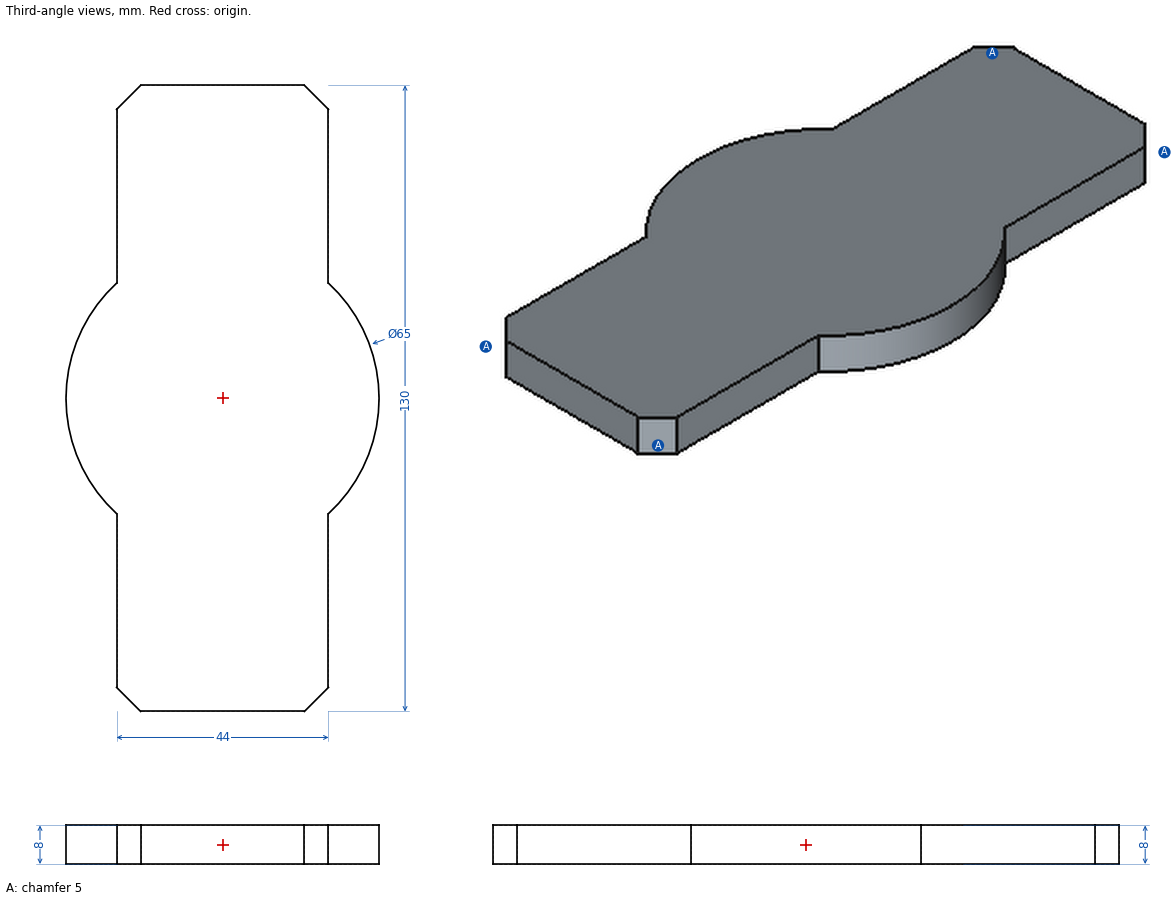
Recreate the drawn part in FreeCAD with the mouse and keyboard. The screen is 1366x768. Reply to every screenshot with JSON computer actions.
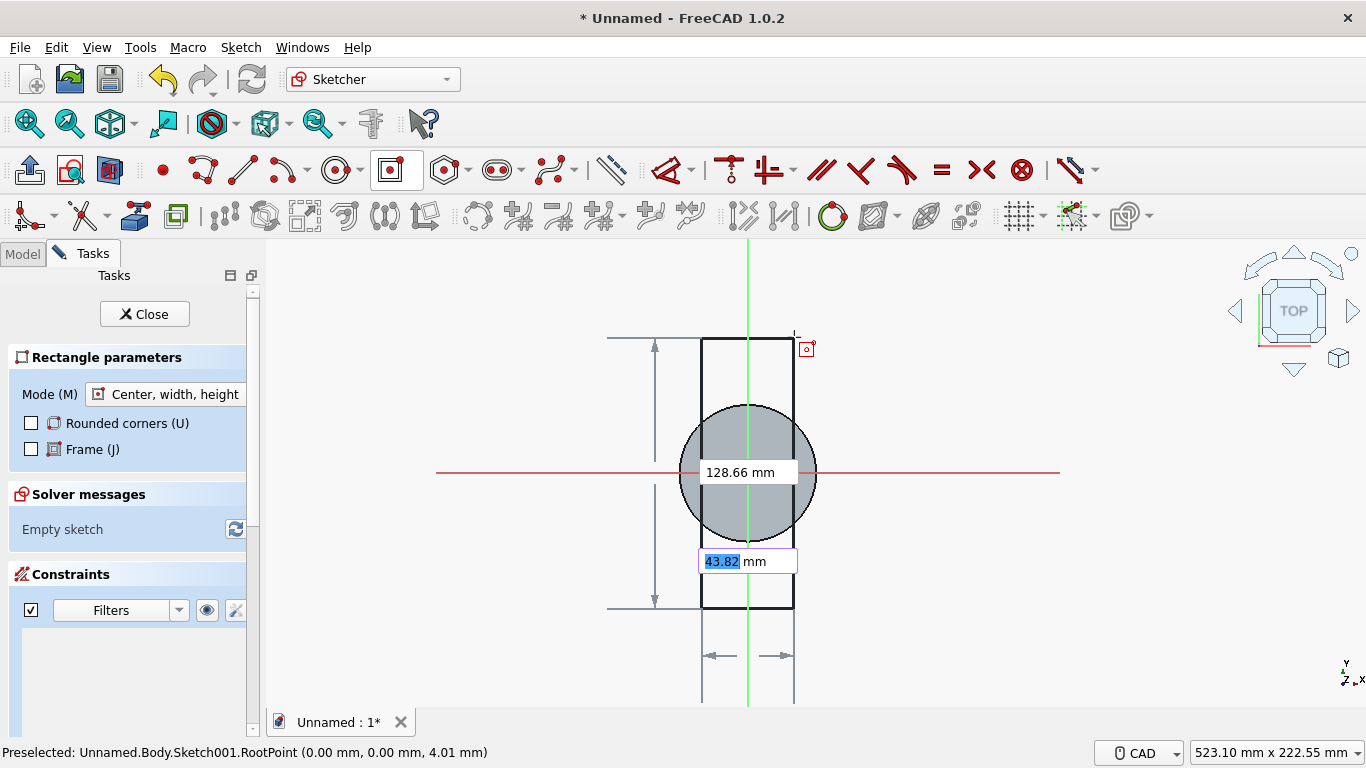
{"action": "type", "text": "44"}
{"action": "key", "text": "Tab"}
{"action": "type", "text": "130"}
{"action": "key", "text": "Return"}
{"action": "key", "text": "Escape"}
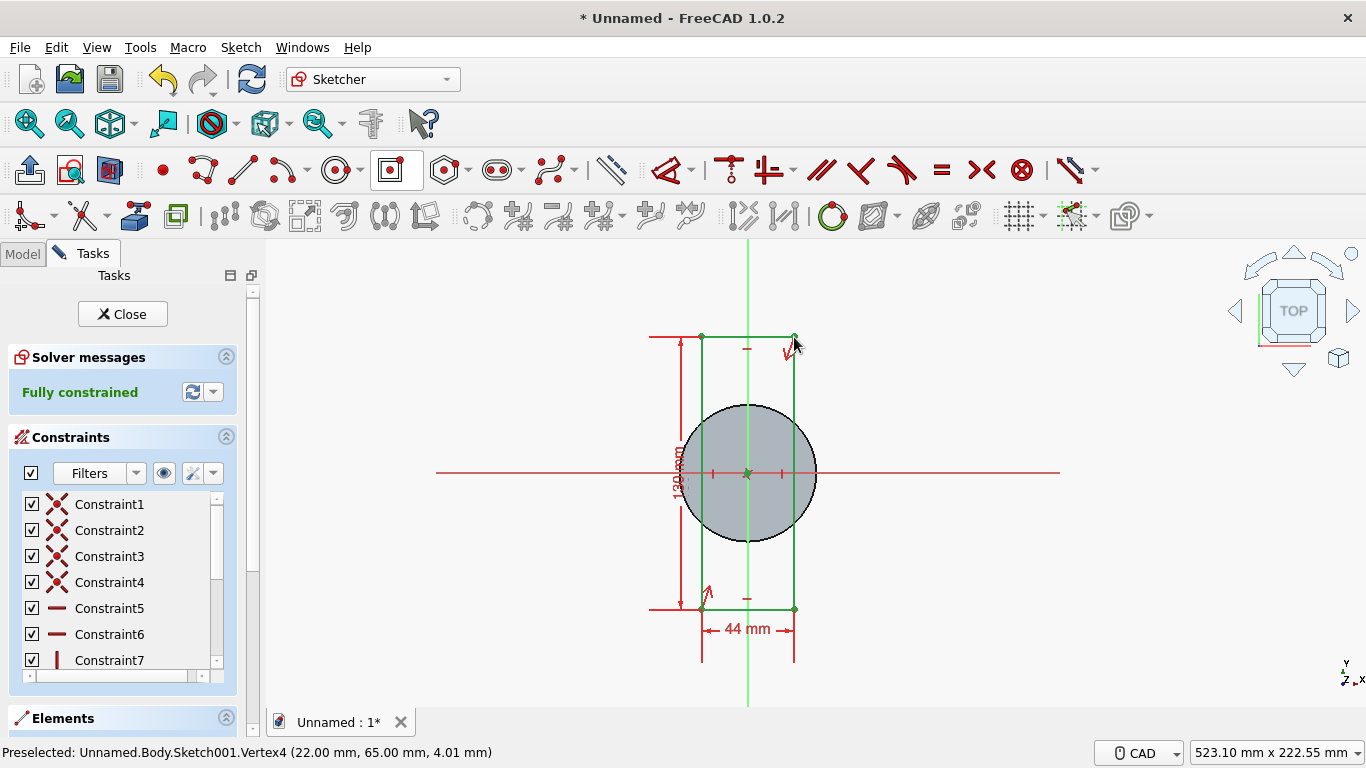
{"action": "left_click", "coordinate": [123, 314]}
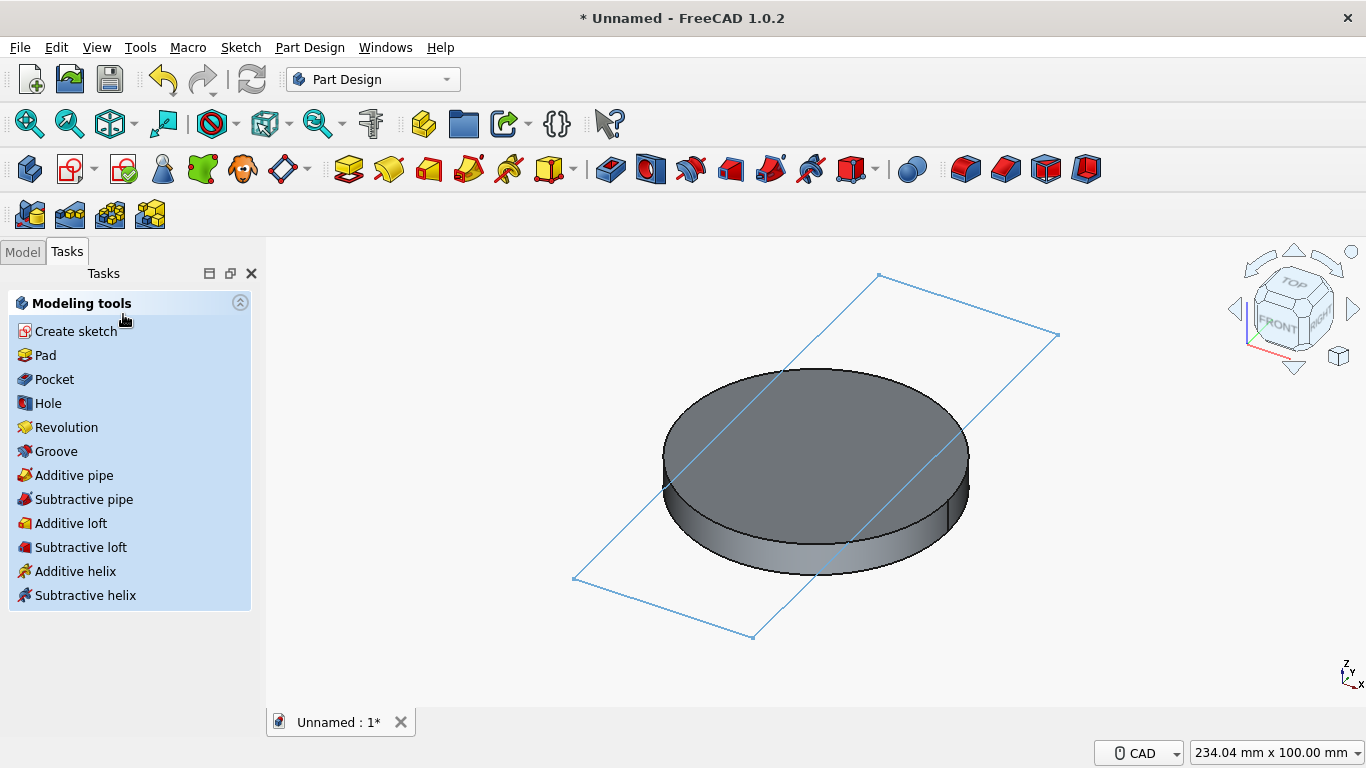
{"action": "left_click", "coordinate": [350, 170]}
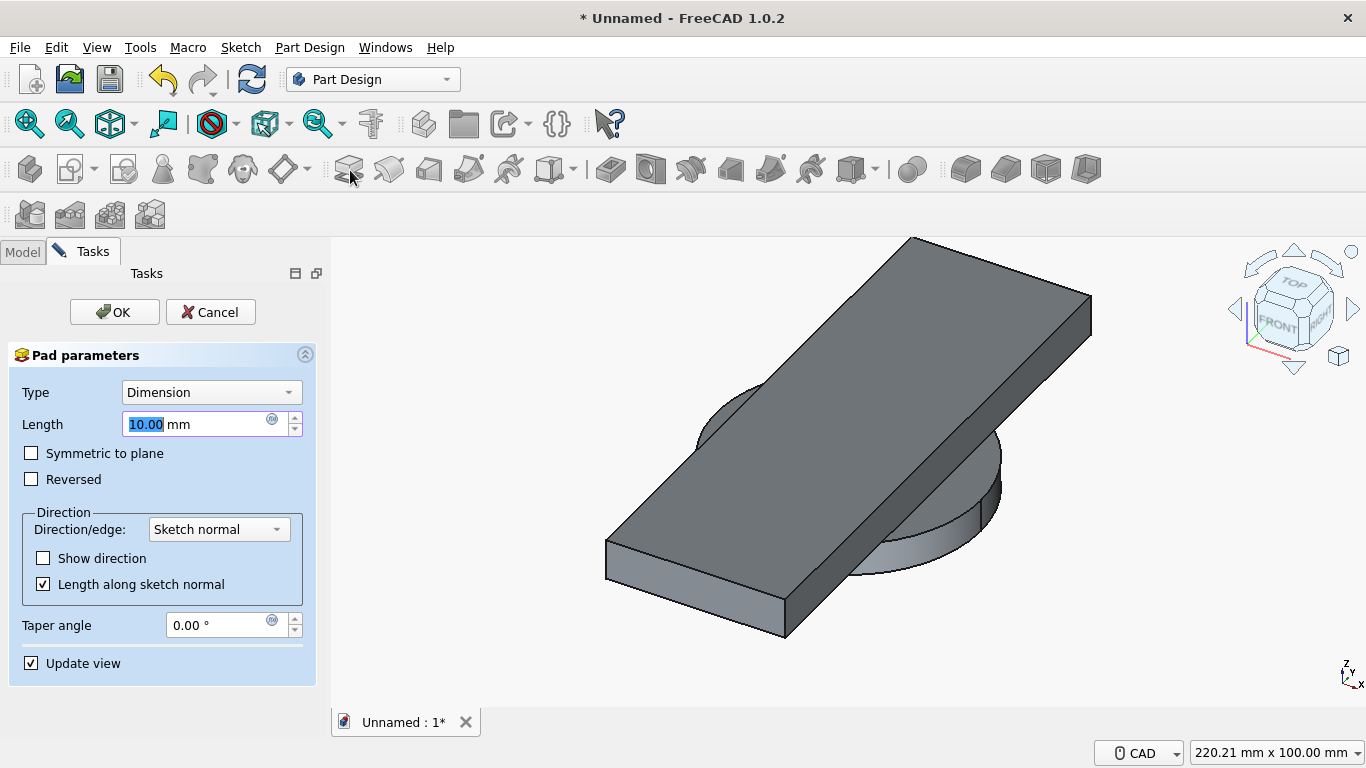
{"action": "type", "text": "8"}
{"action": "key", "text": "Tab"}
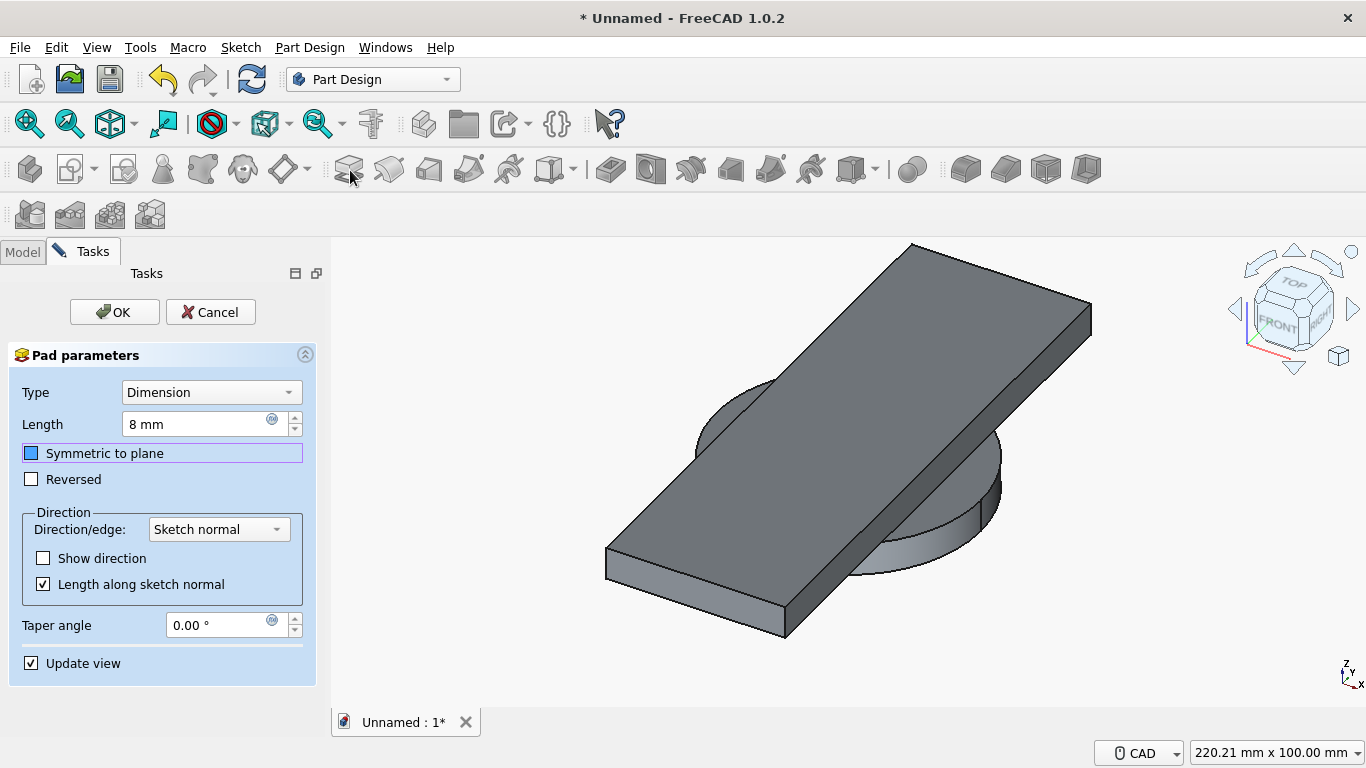
{"action": "left_click", "coordinate": [30, 479]}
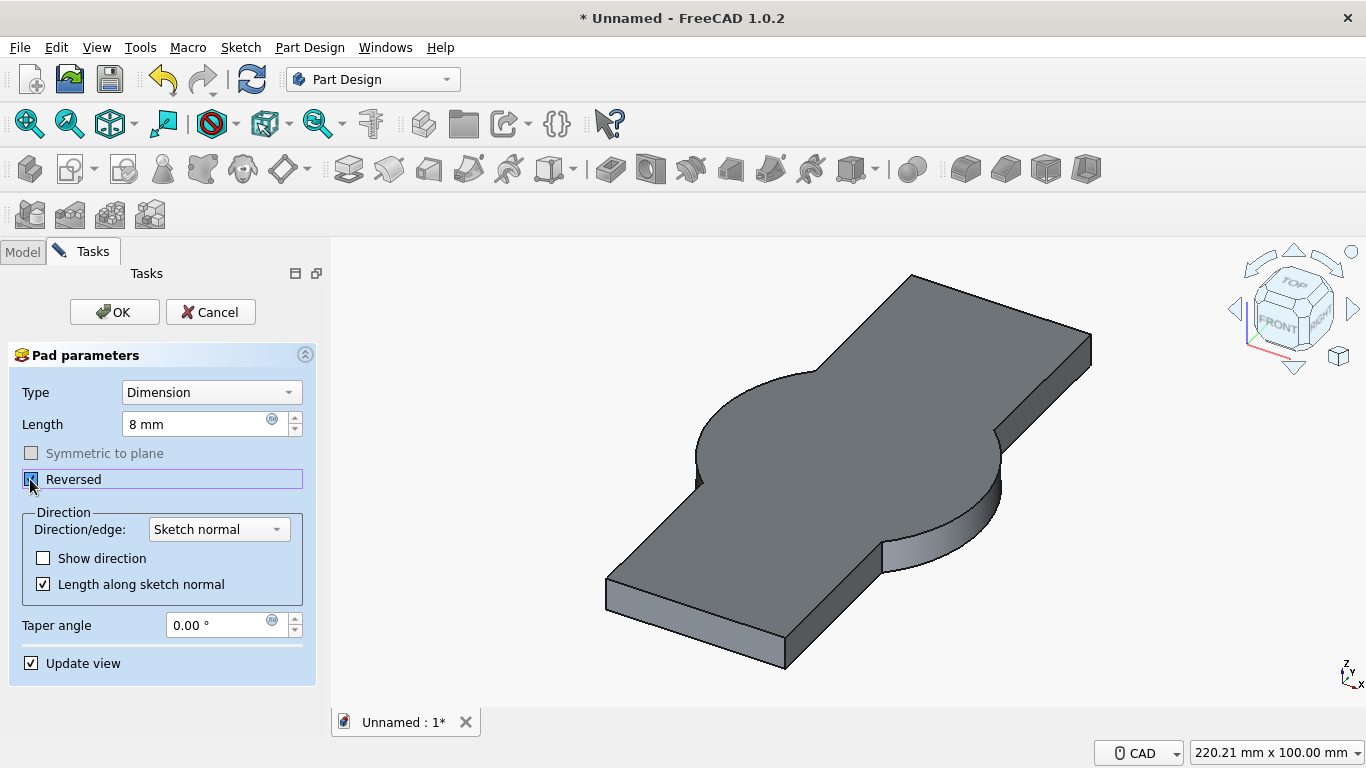
{"action": "left_click", "coordinate": [115, 312]}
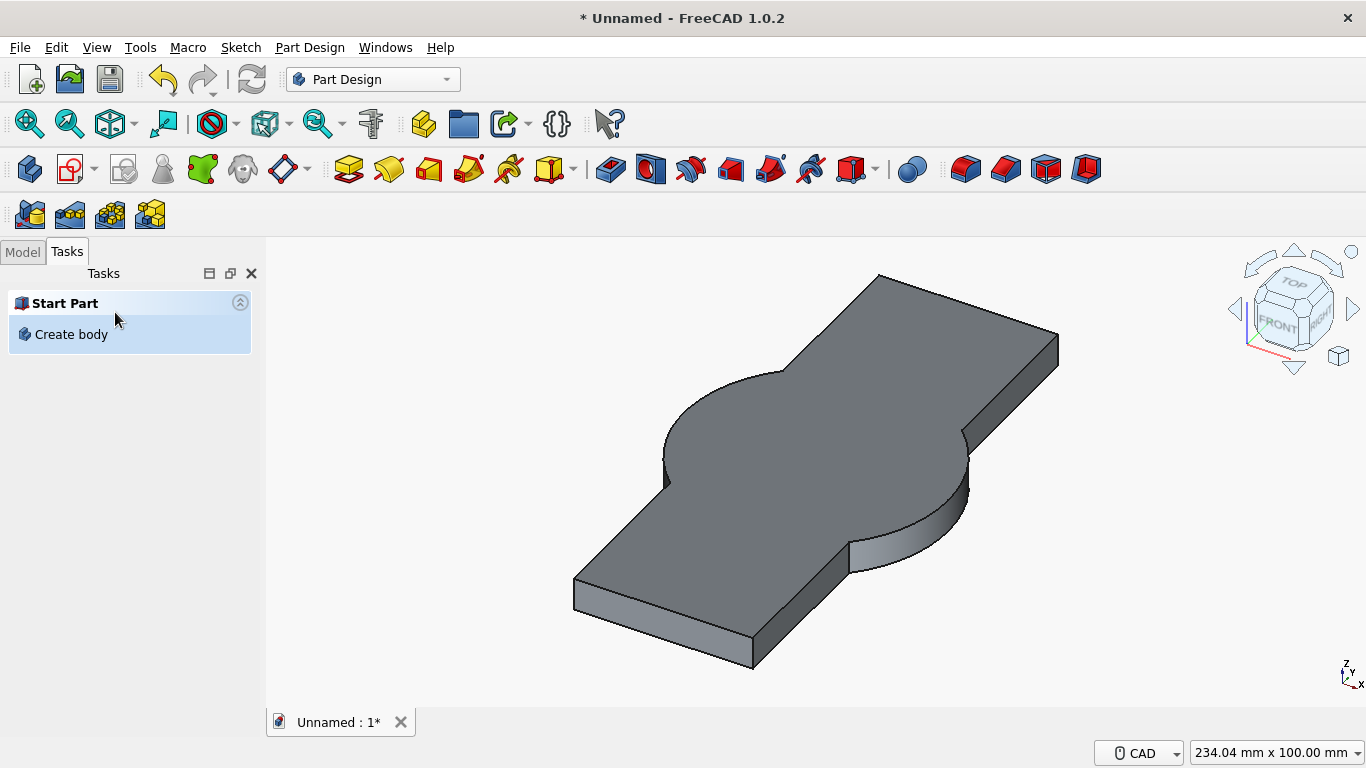
{"action": "left_click", "coordinate": [753, 652]}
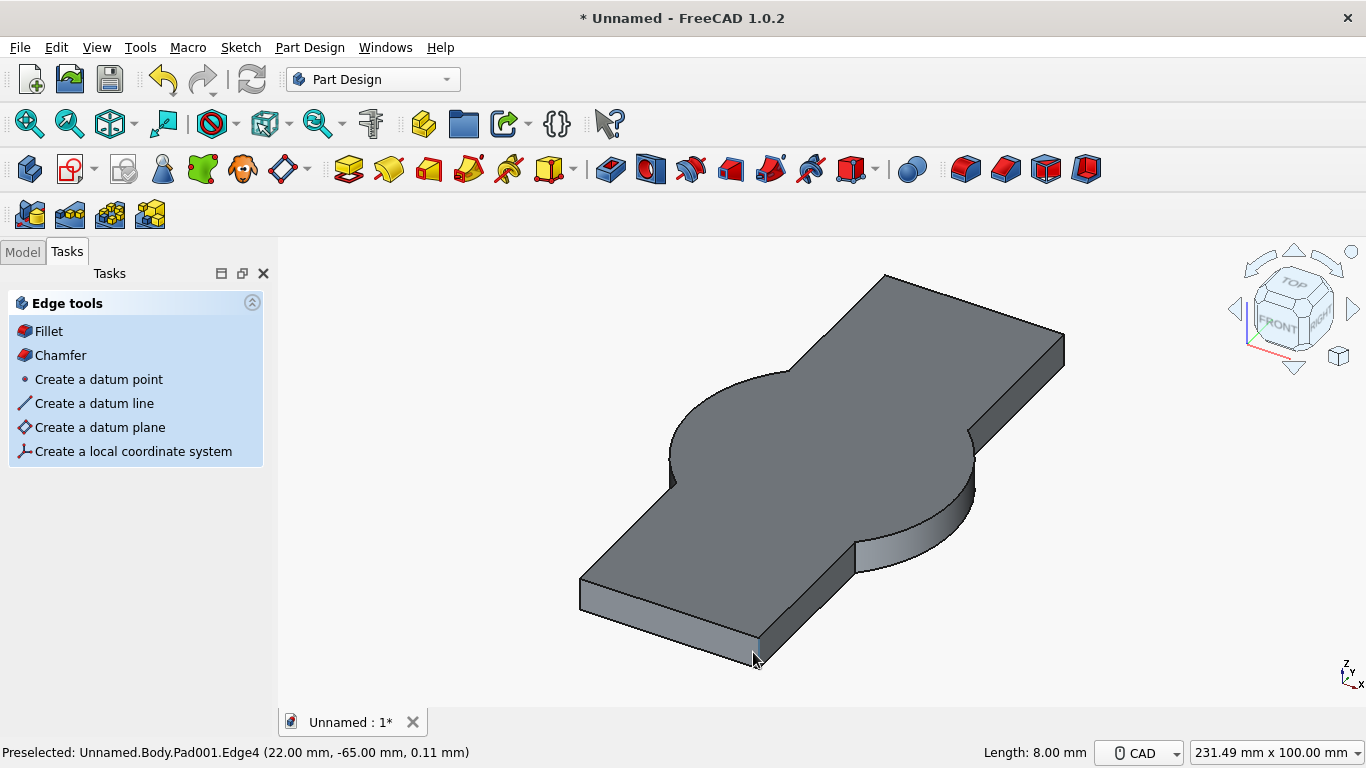
{"action": "key", "text": "0"}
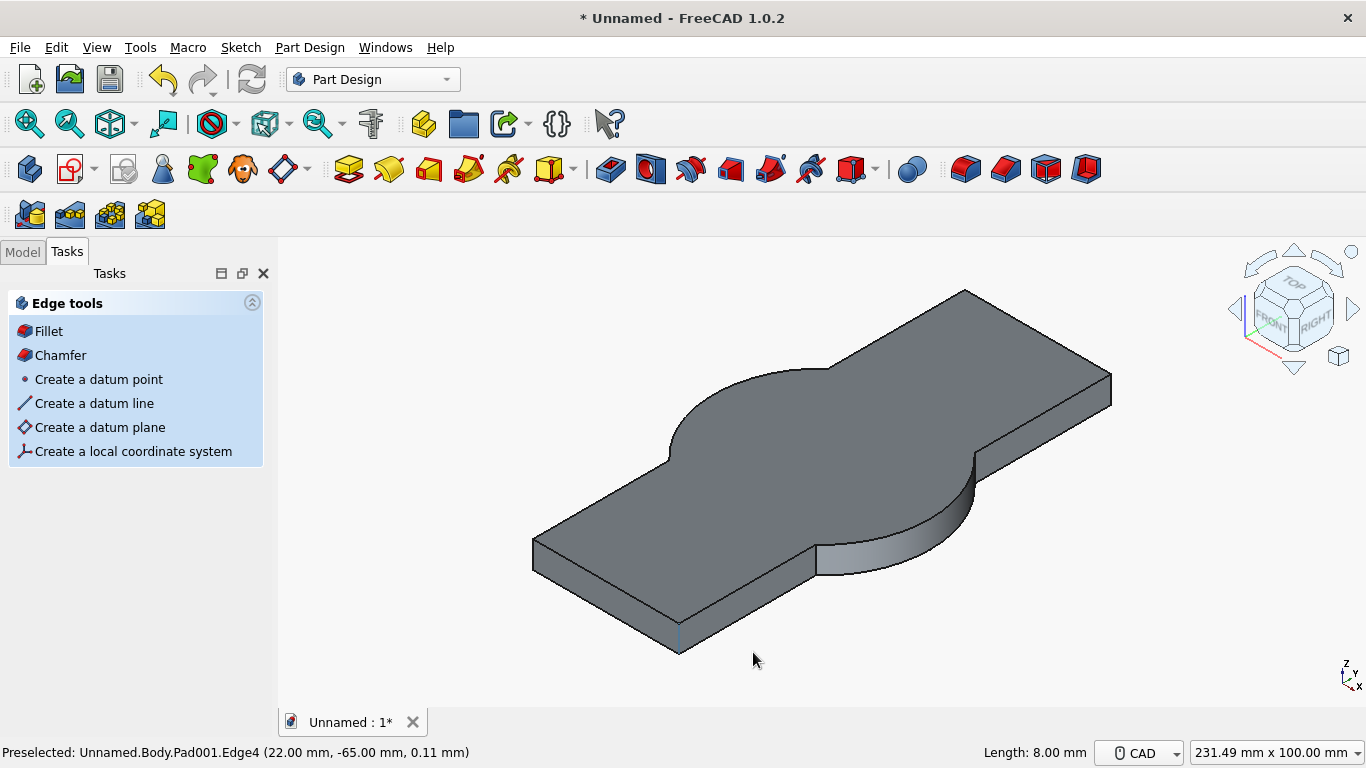
{"action": "key", "text": "2"}